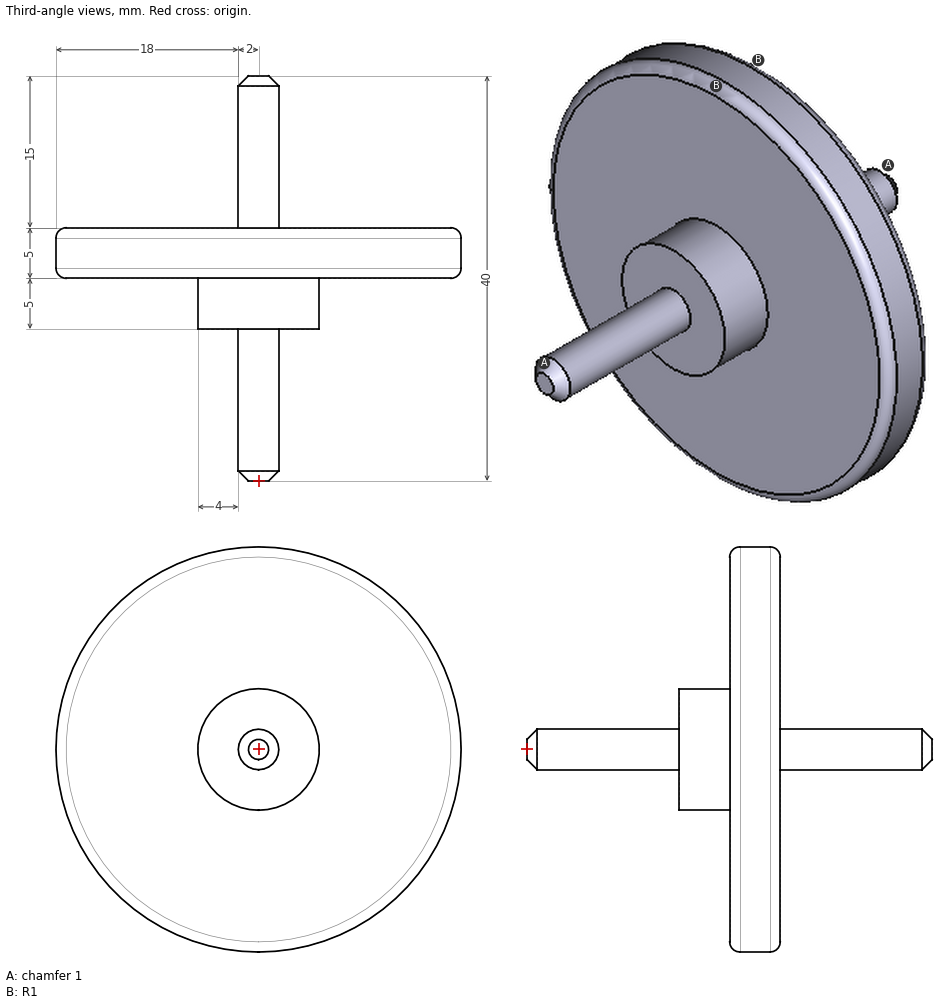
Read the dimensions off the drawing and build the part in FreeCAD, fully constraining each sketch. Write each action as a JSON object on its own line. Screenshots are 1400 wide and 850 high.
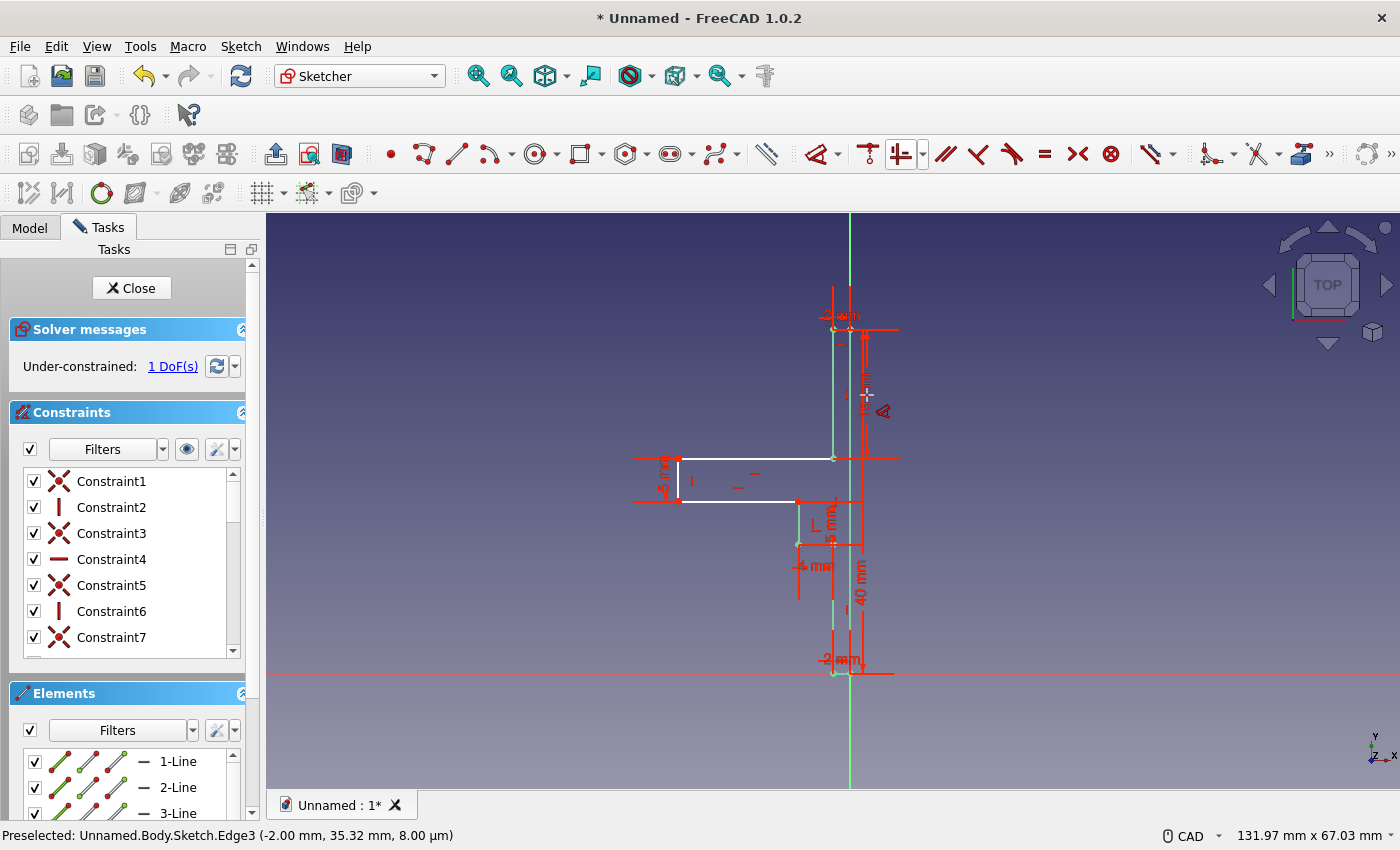
{"action": "left_click", "coordinate": [787, 459]}
{"action": "left_click", "coordinate": [756, 425]}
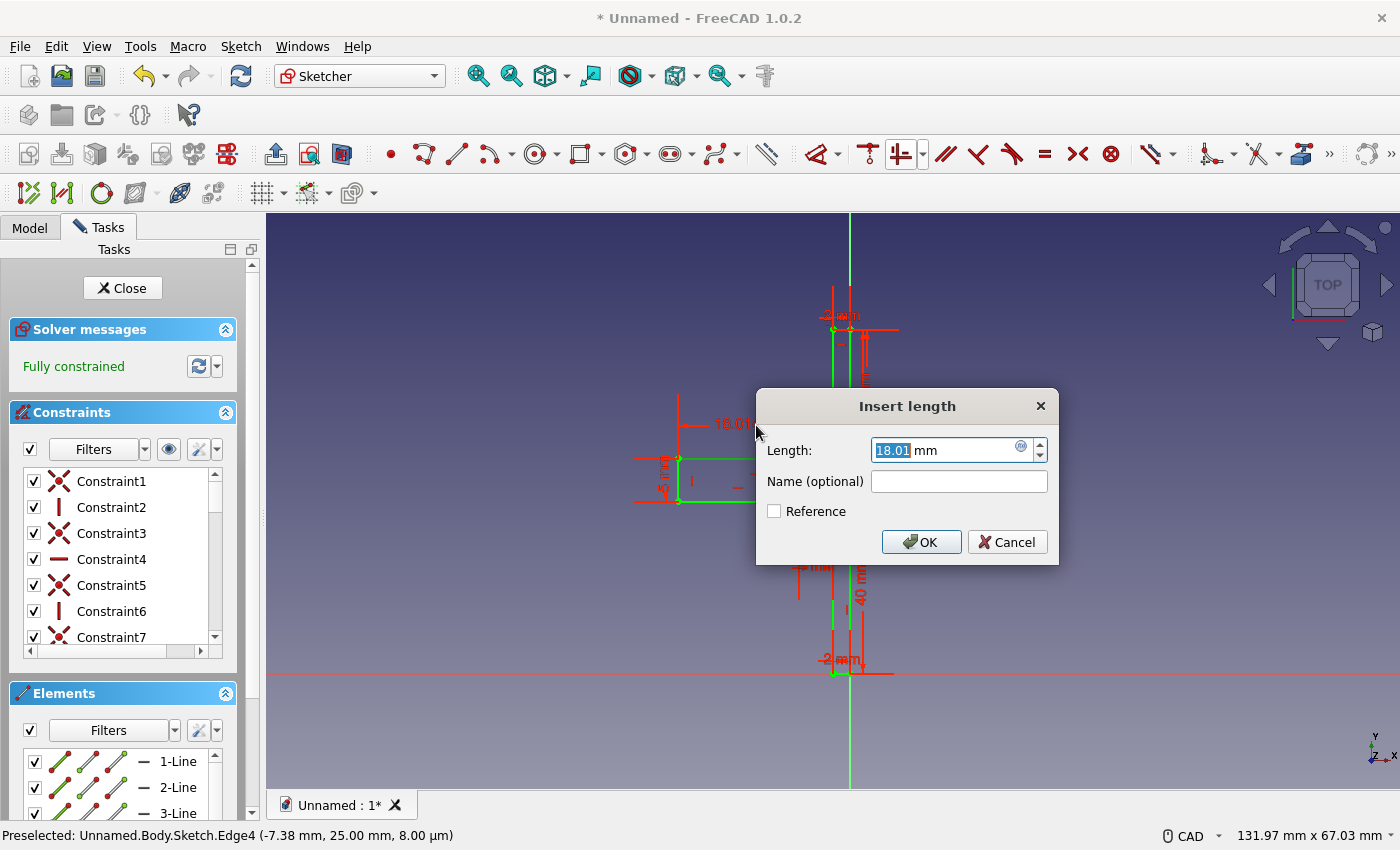
{"action": "type", "text": "18"}
{"action": "key", "text": "Return"}
{"action": "key", "text": "Escape"}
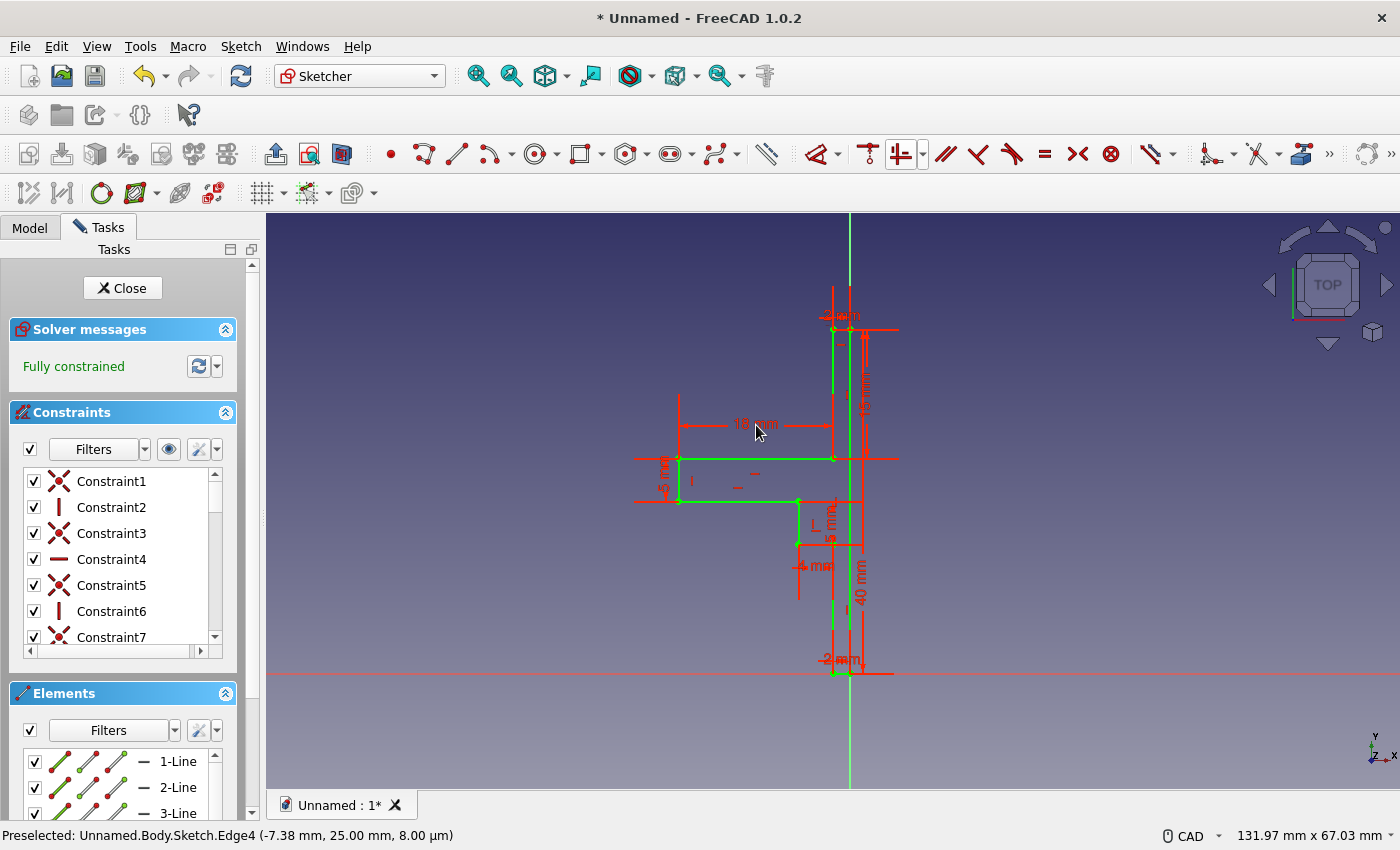
{"action": "left_click", "coordinate": [123, 288]}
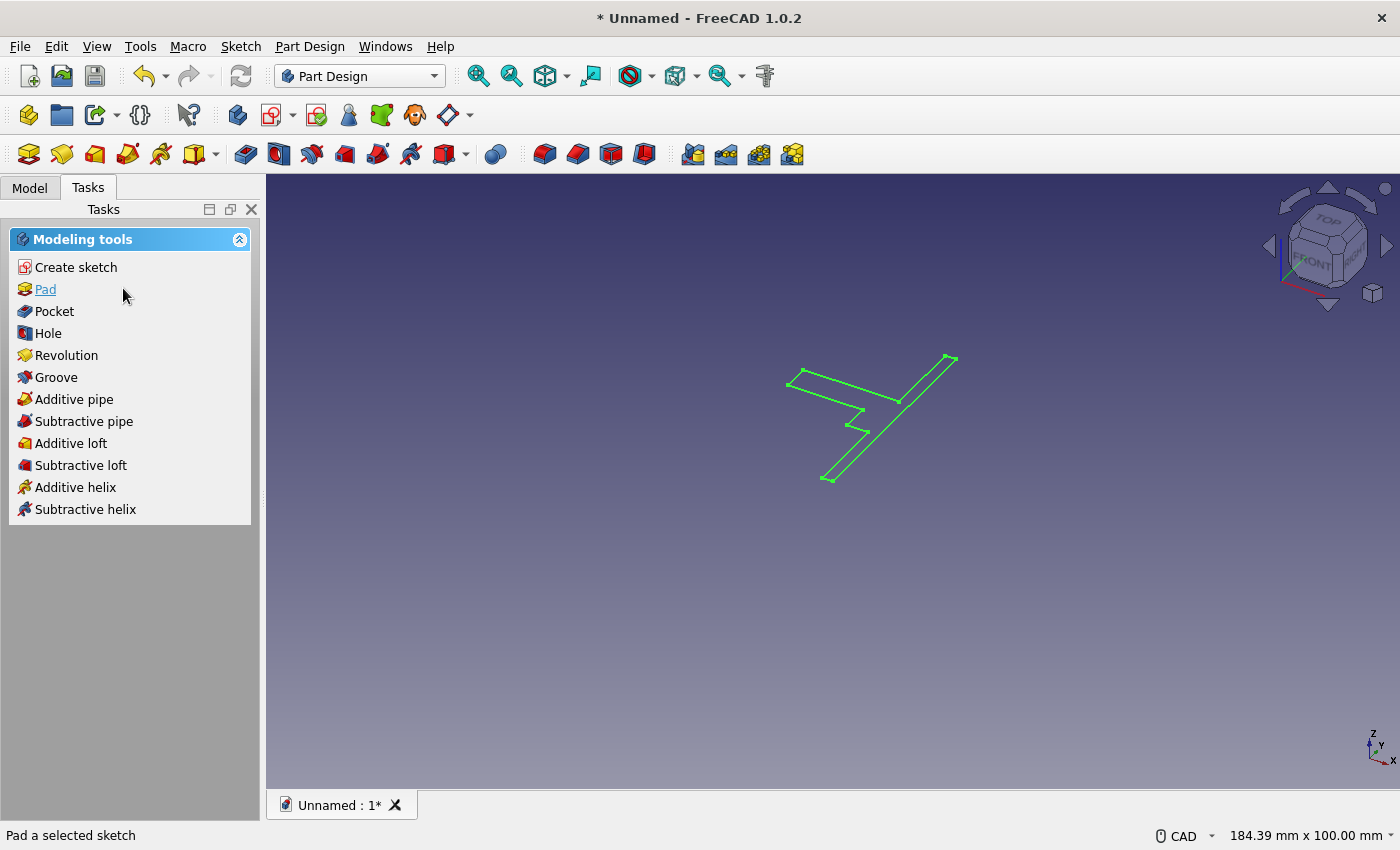
{"action": "left_click", "coordinate": [62, 154]}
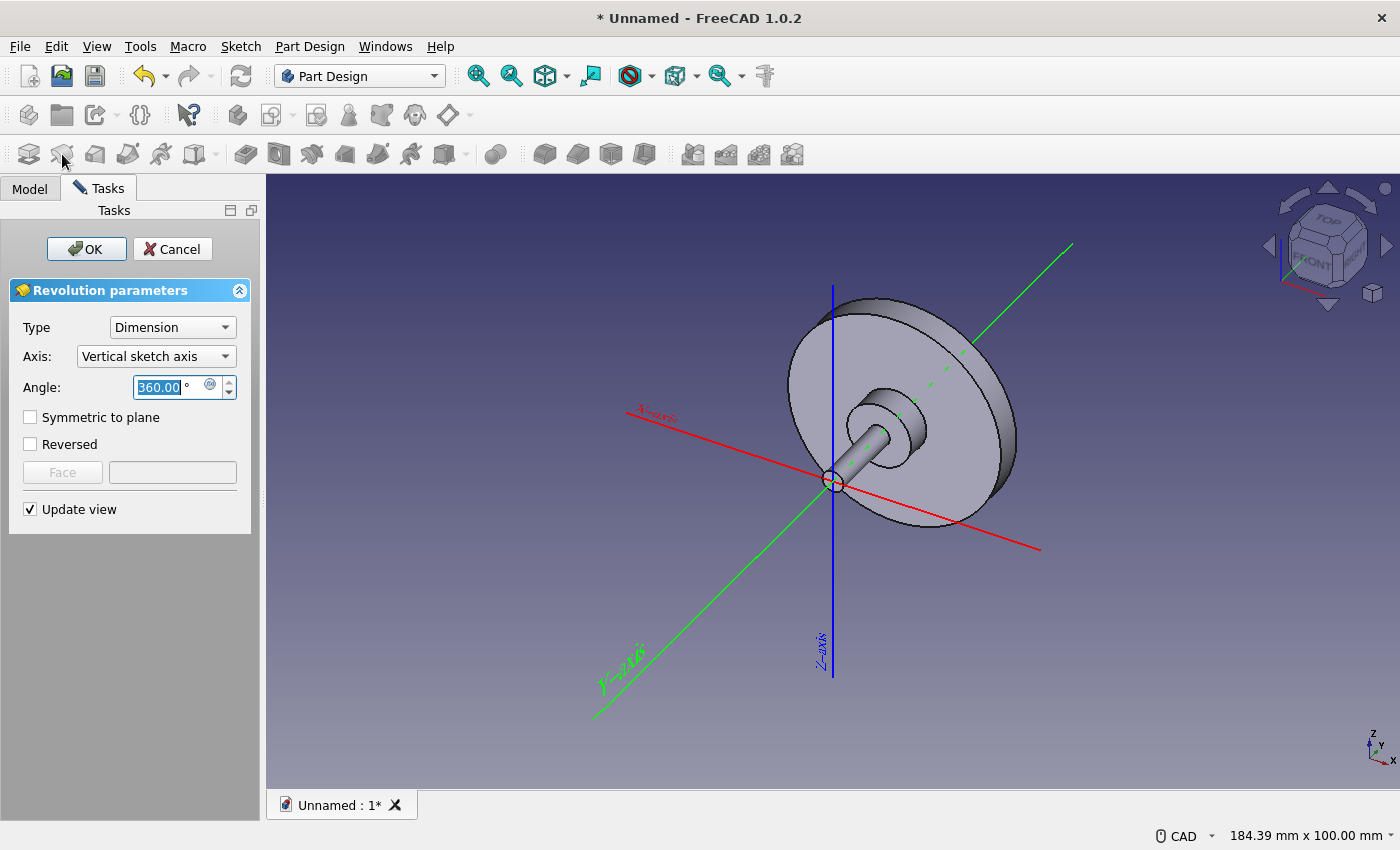
{"action": "left_click", "coordinate": [87, 249]}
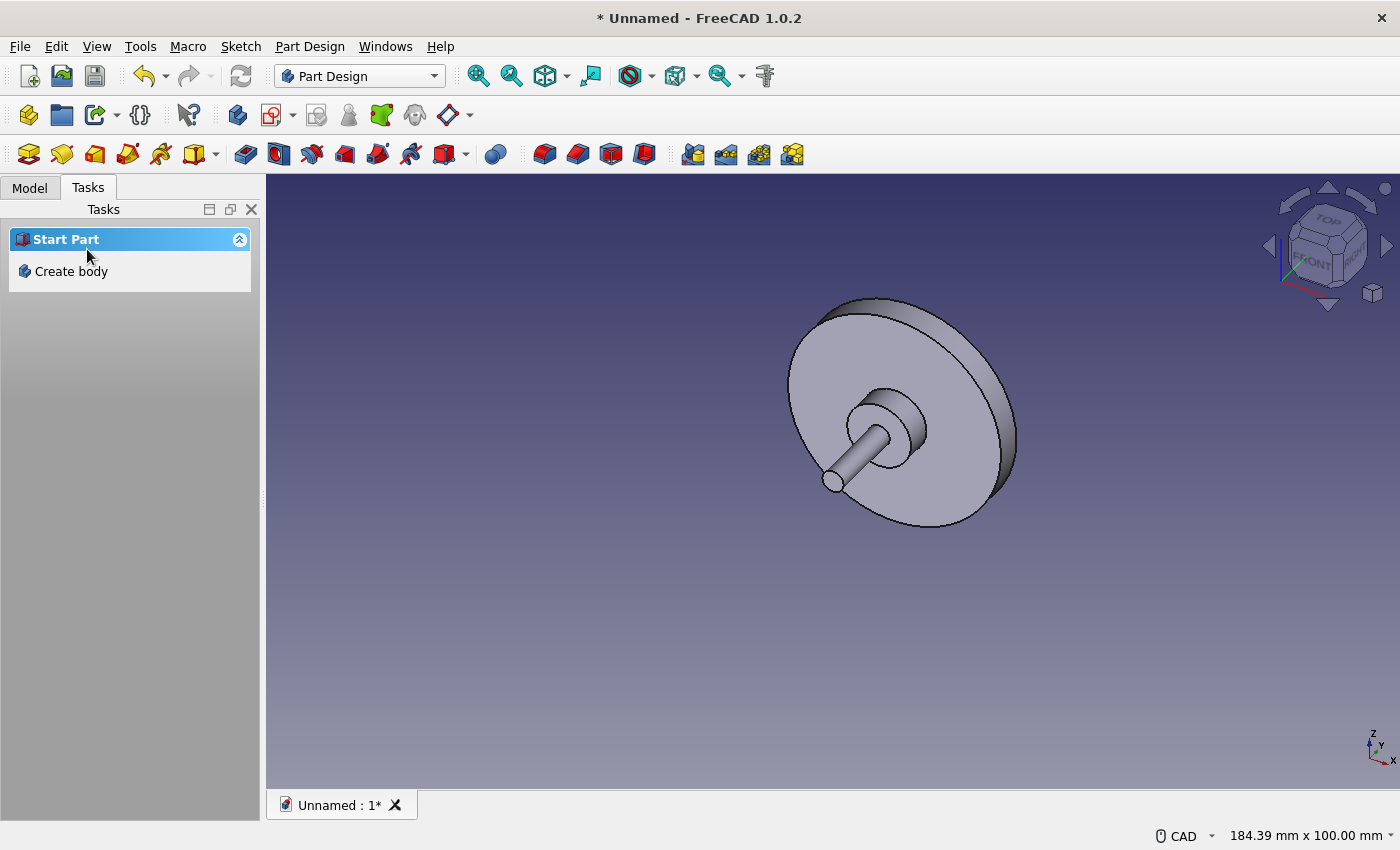
{"action": "left_click", "coordinate": [844, 484]}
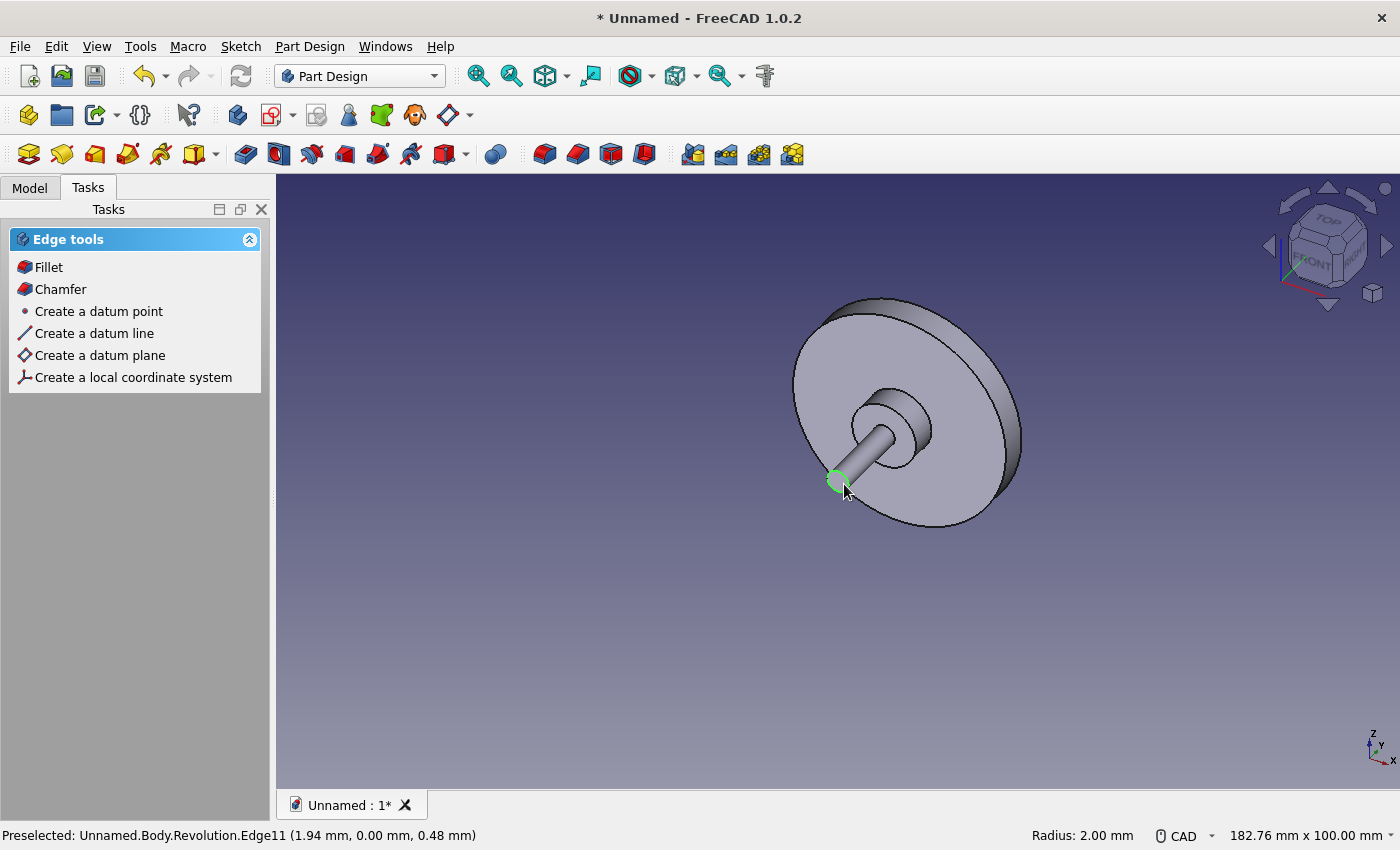
{"action": "key", "text": "0"}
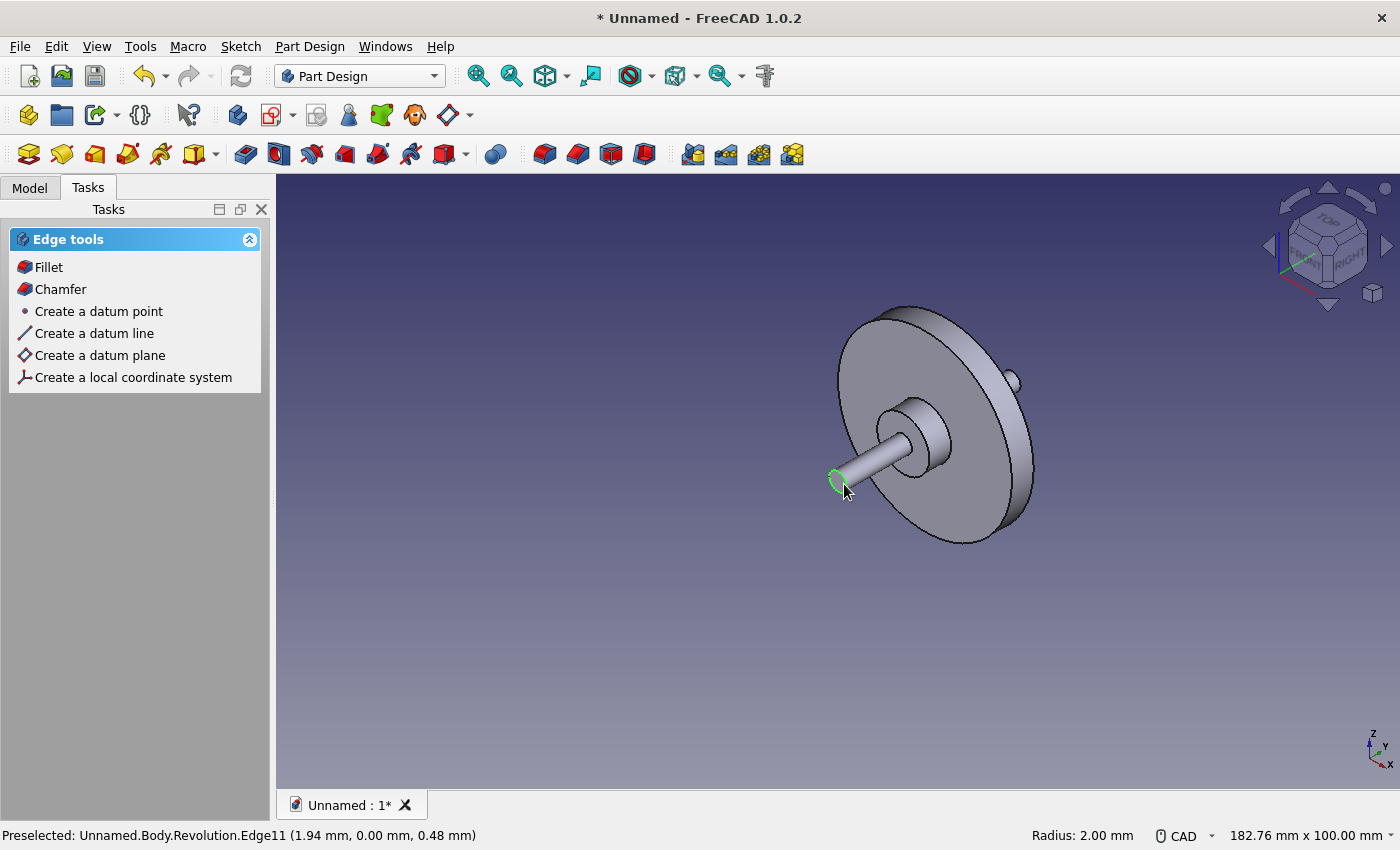
{"action": "left_click", "coordinate": [1021, 385], "text": "ctrl"}